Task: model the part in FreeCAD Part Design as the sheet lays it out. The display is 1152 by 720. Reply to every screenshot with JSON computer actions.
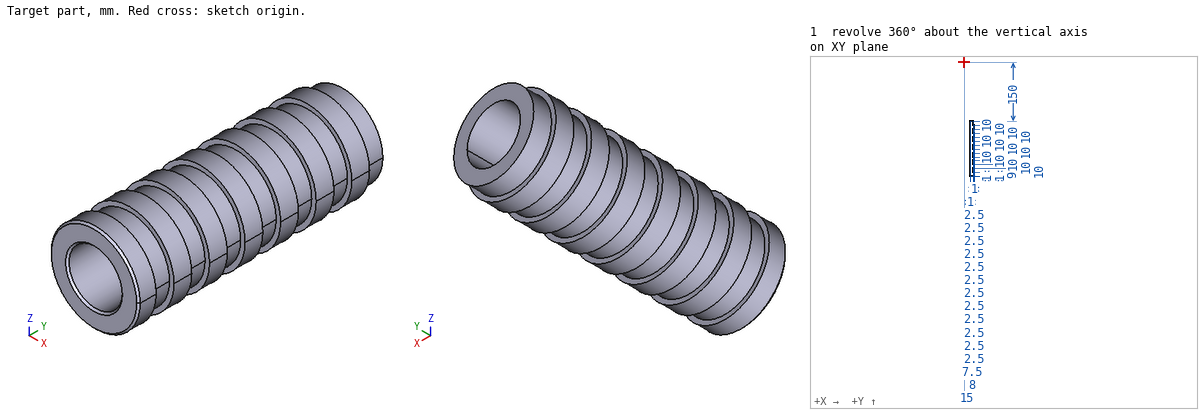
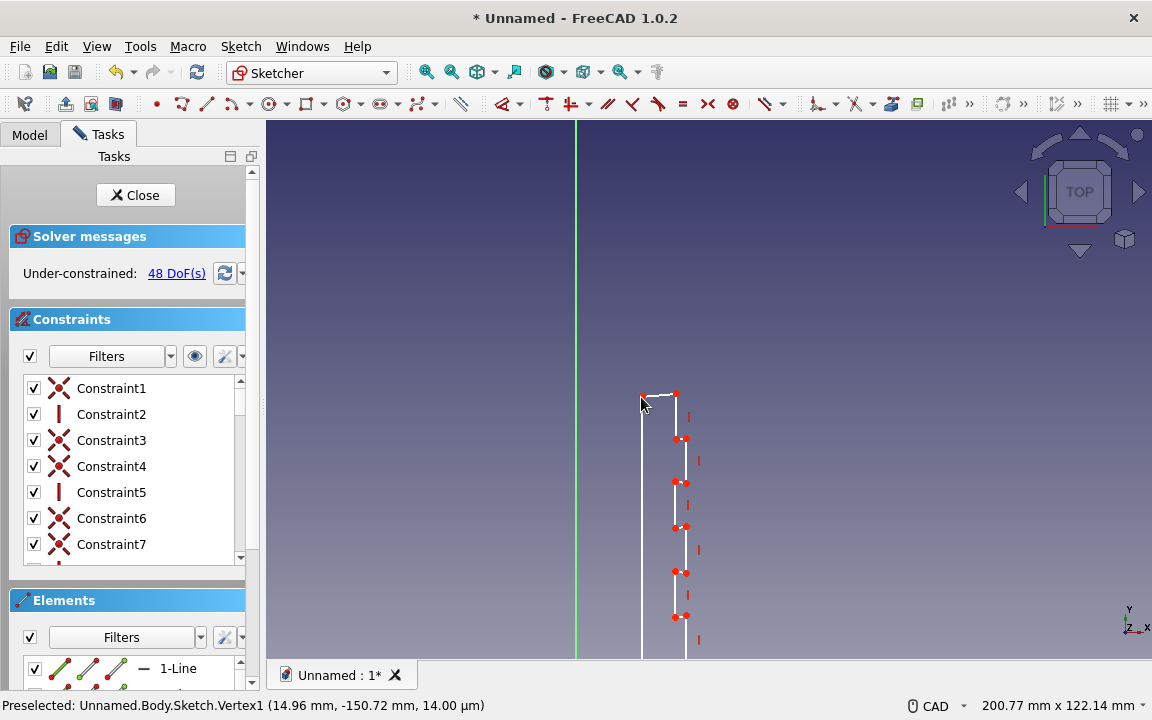
{"action": "scroll", "coordinate": [652, 396], "scroll_direction": "up", "scroll_amount": 2}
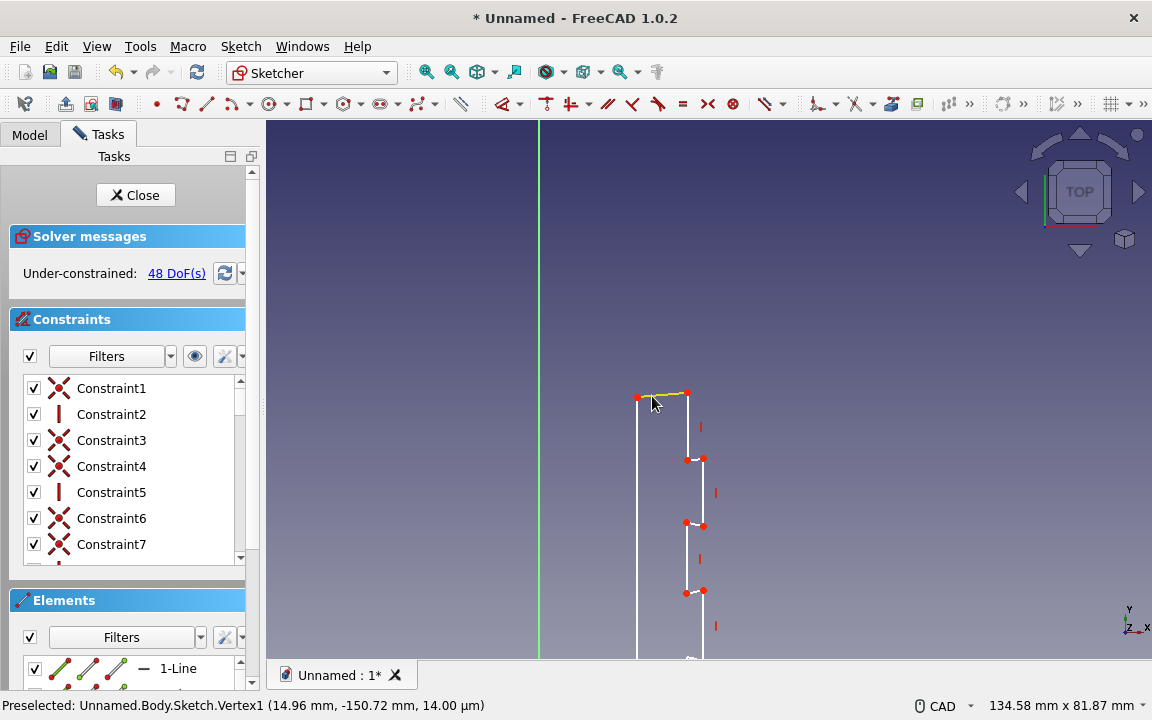
{"action": "left_click", "coordinate": [652, 396]}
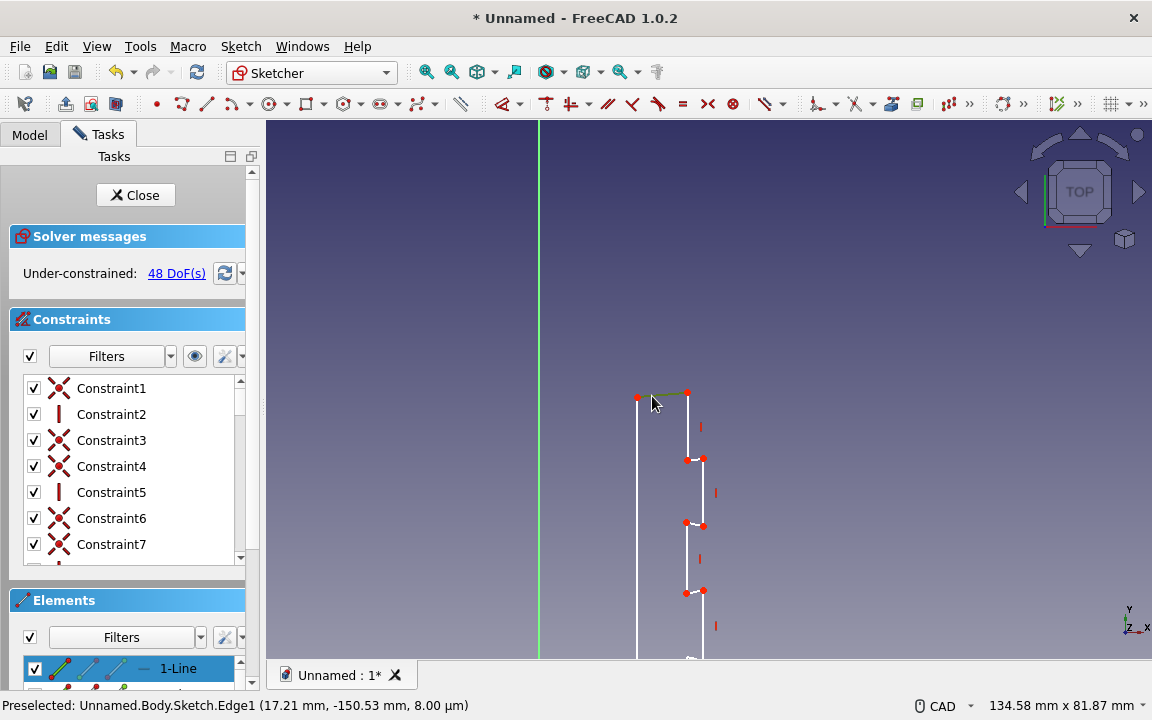
{"action": "key", "text": "h"}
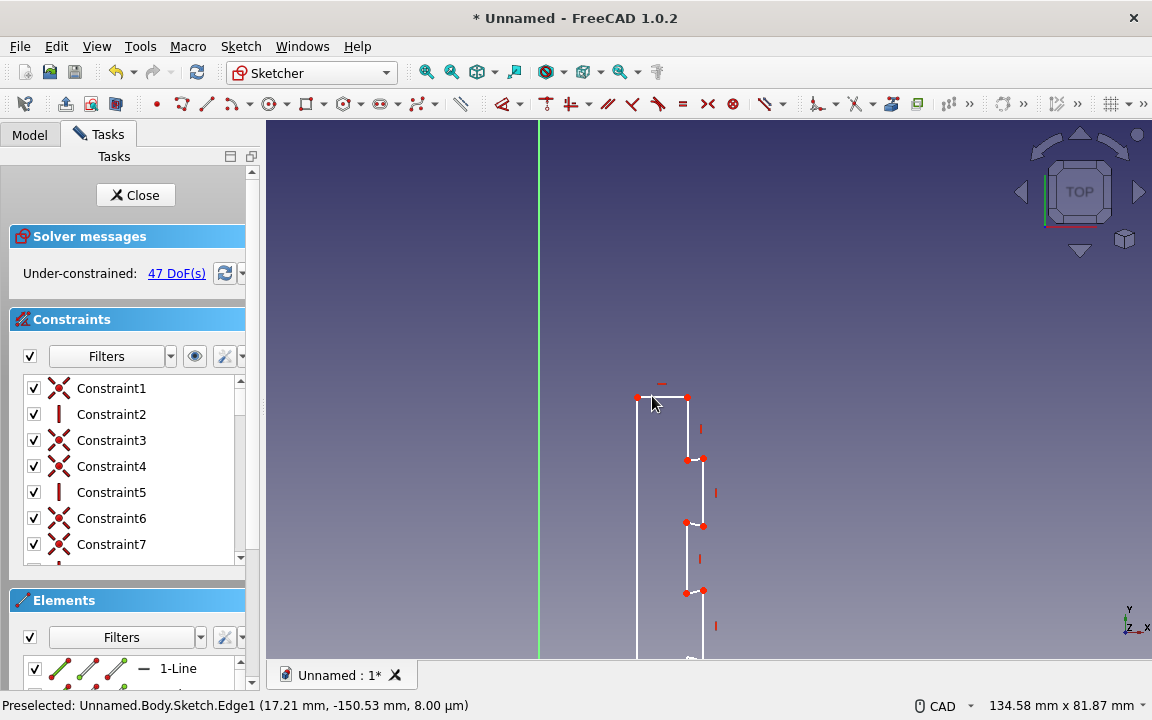
{"action": "scroll", "coordinate": [696, 460], "scroll_direction": "up", "scroll_amount": 4}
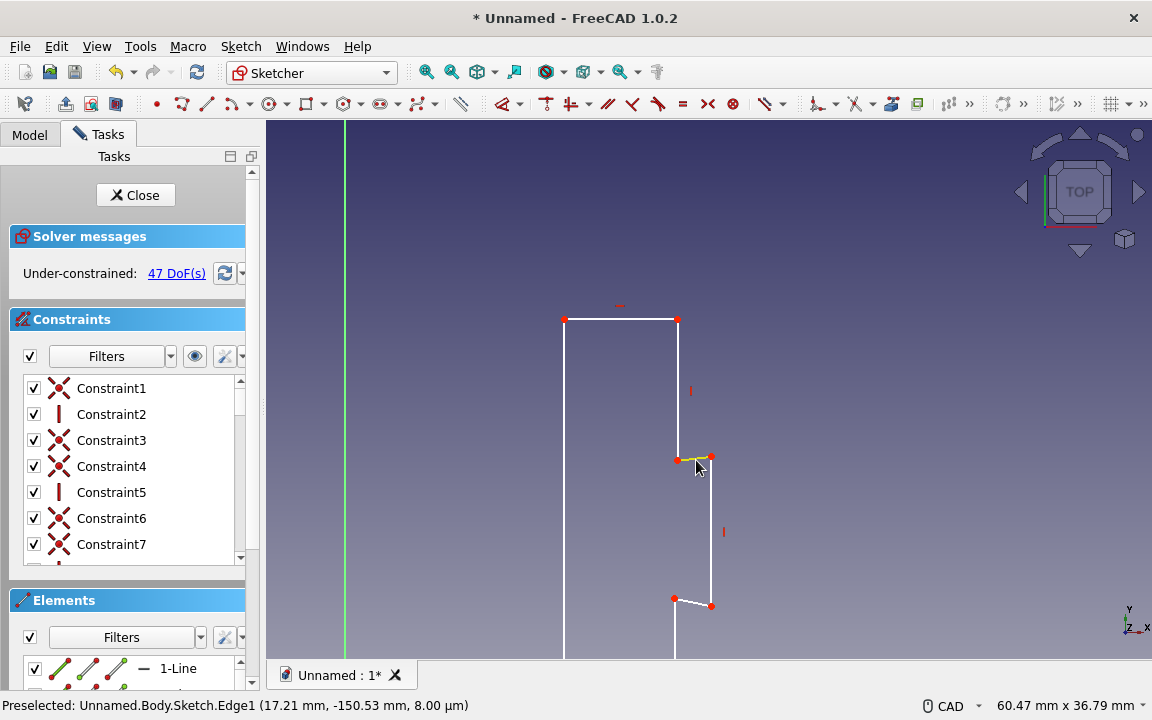
{"action": "left_click", "coordinate": [694, 459]}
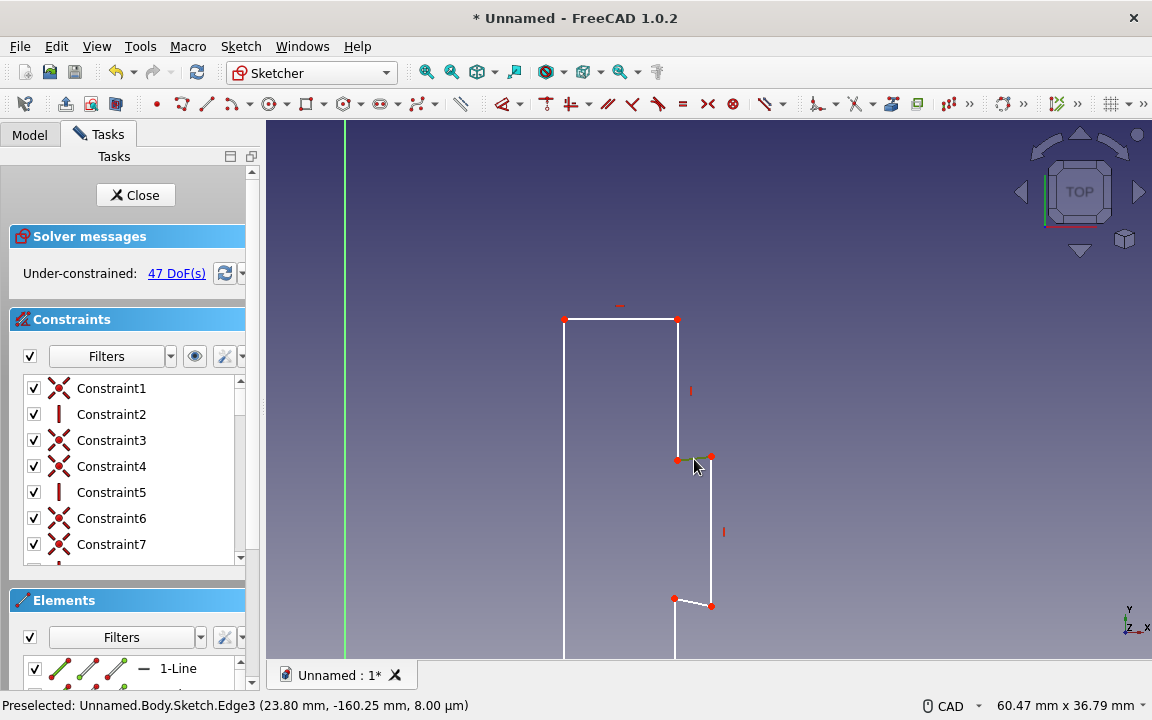
{"action": "left_click", "coordinate": [588, 104]}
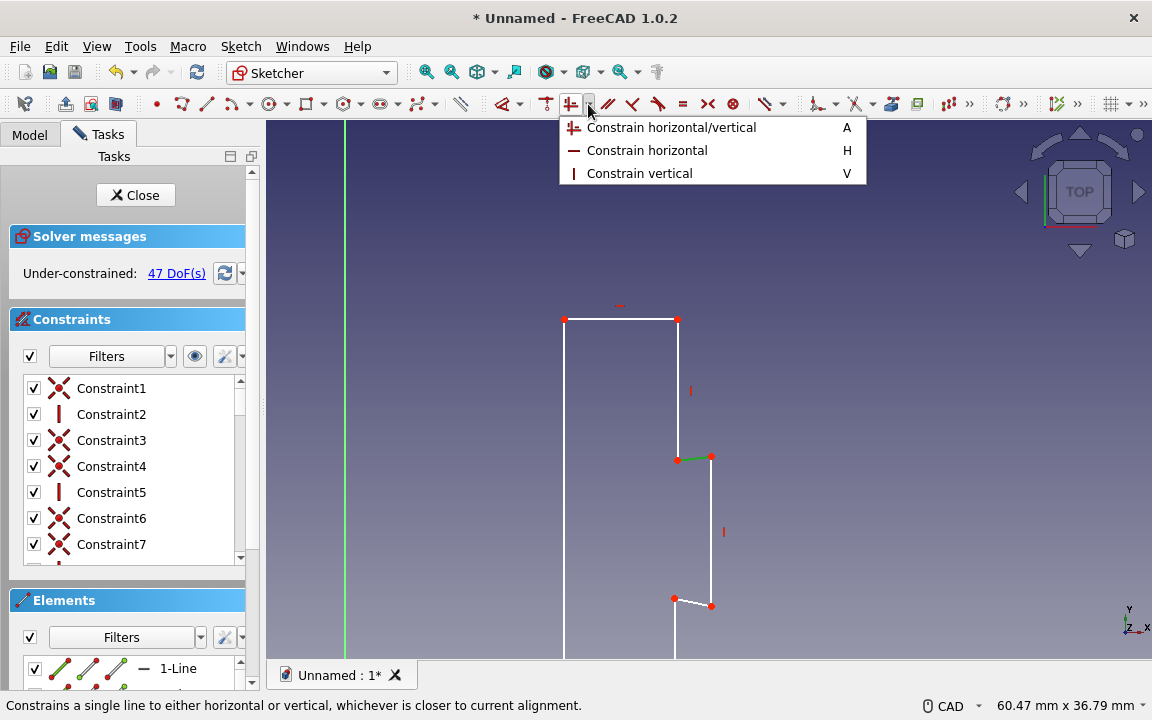
{"action": "left_click", "coordinate": [713, 150]}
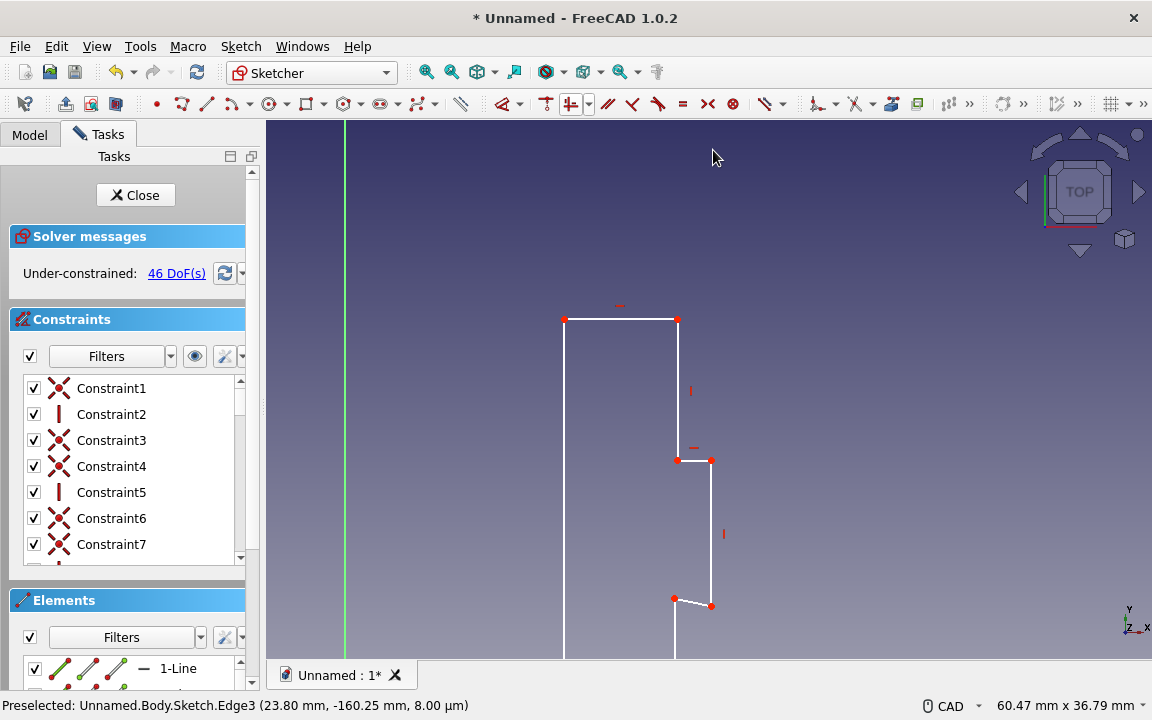
{"action": "left_click", "coordinate": [700, 604]}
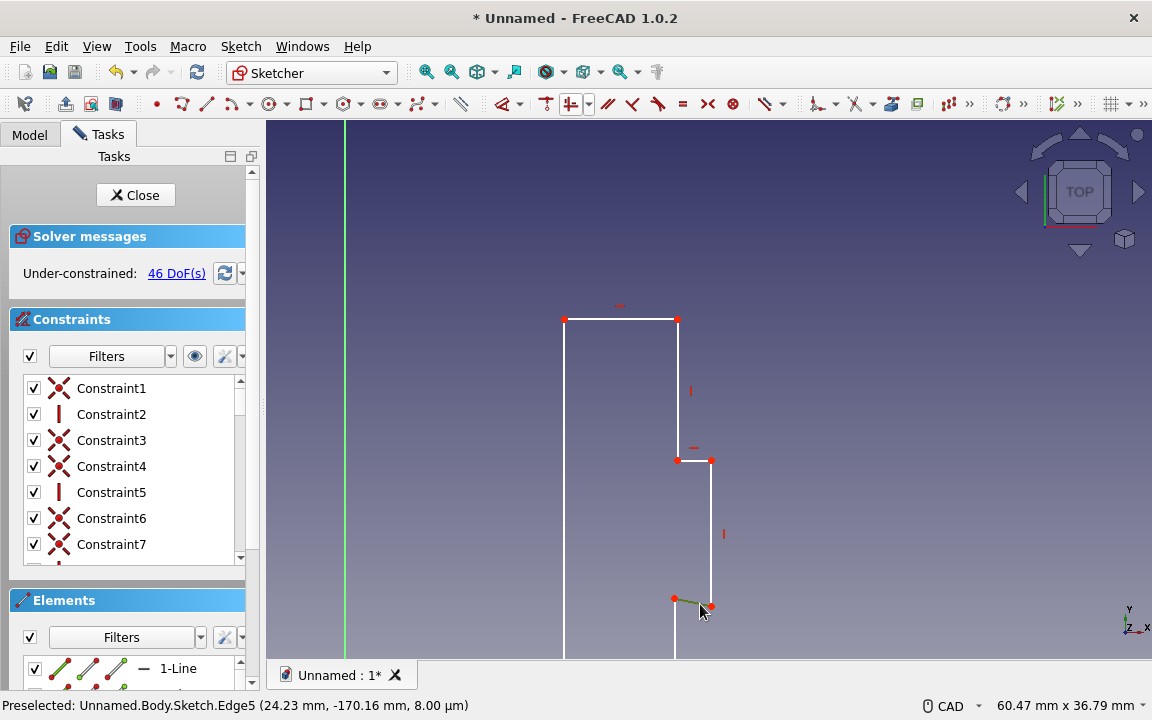
{"action": "key", "text": "h"}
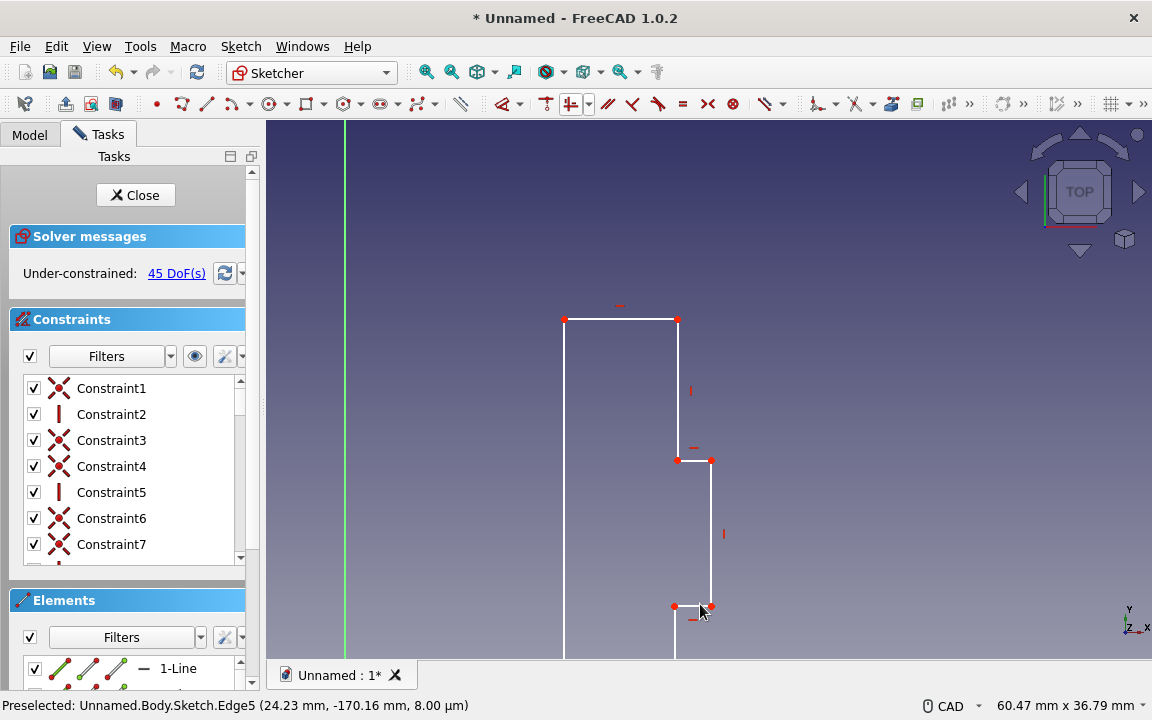
{"action": "scroll", "coordinate": [650, 402], "scroll_direction": "down", "scroll_amount": 13}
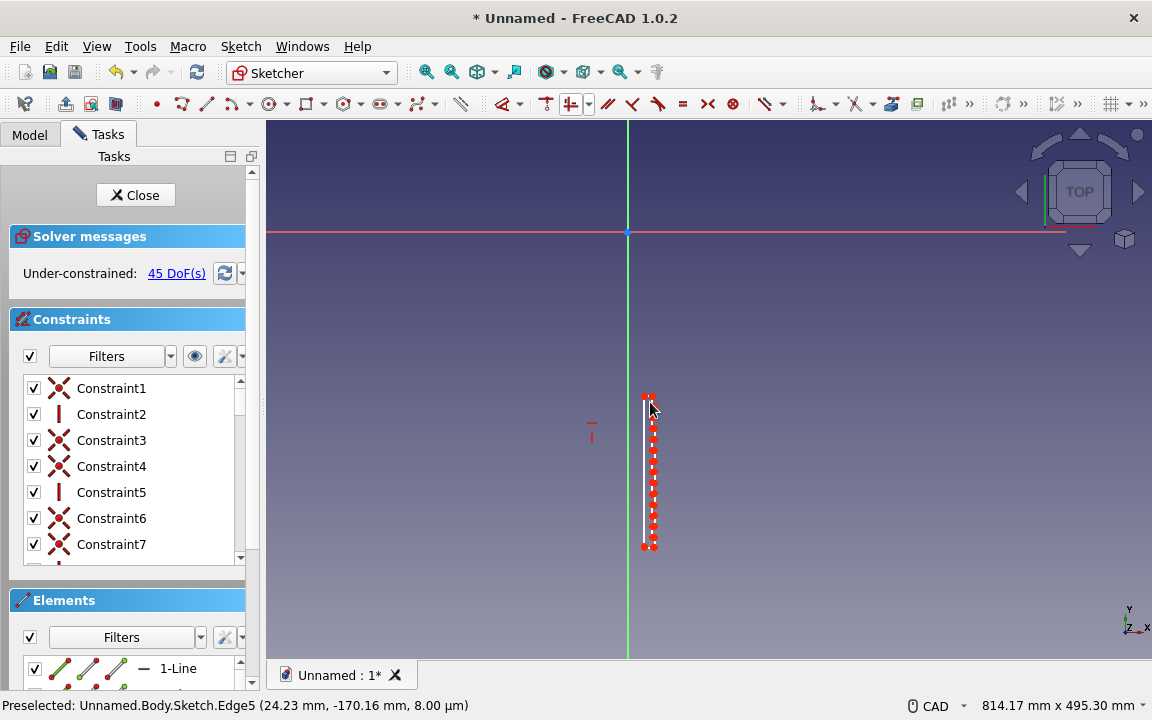
{"action": "scroll", "coordinate": [653, 429], "scroll_direction": "up", "scroll_amount": 14}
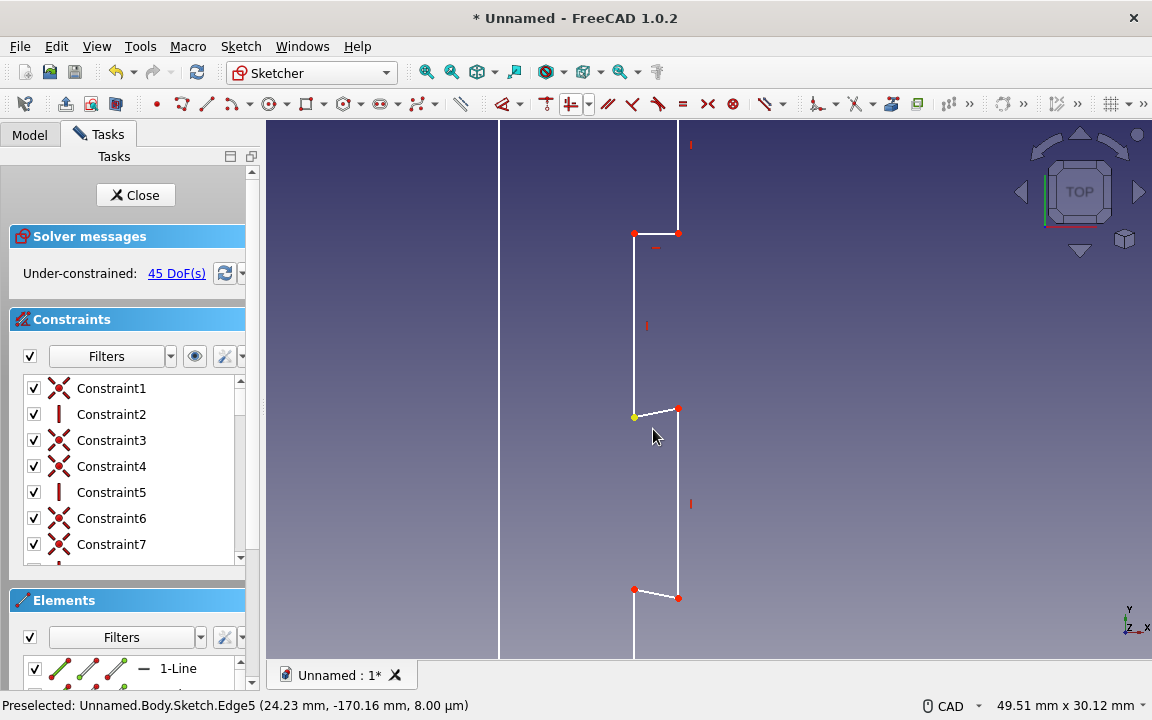
{"action": "left_click", "coordinate": [647, 415]}